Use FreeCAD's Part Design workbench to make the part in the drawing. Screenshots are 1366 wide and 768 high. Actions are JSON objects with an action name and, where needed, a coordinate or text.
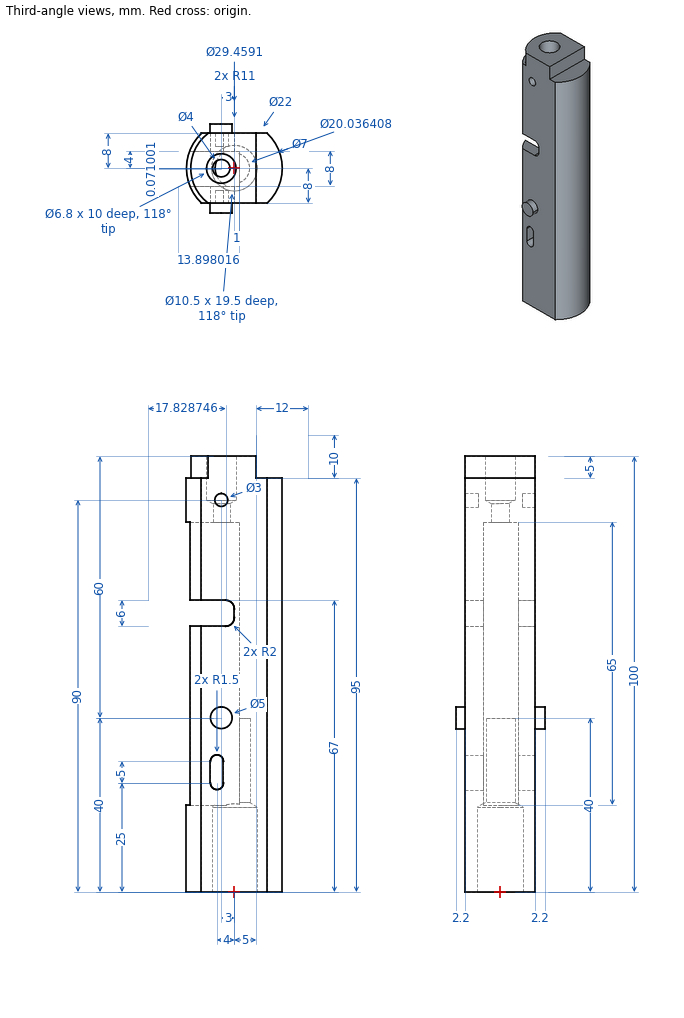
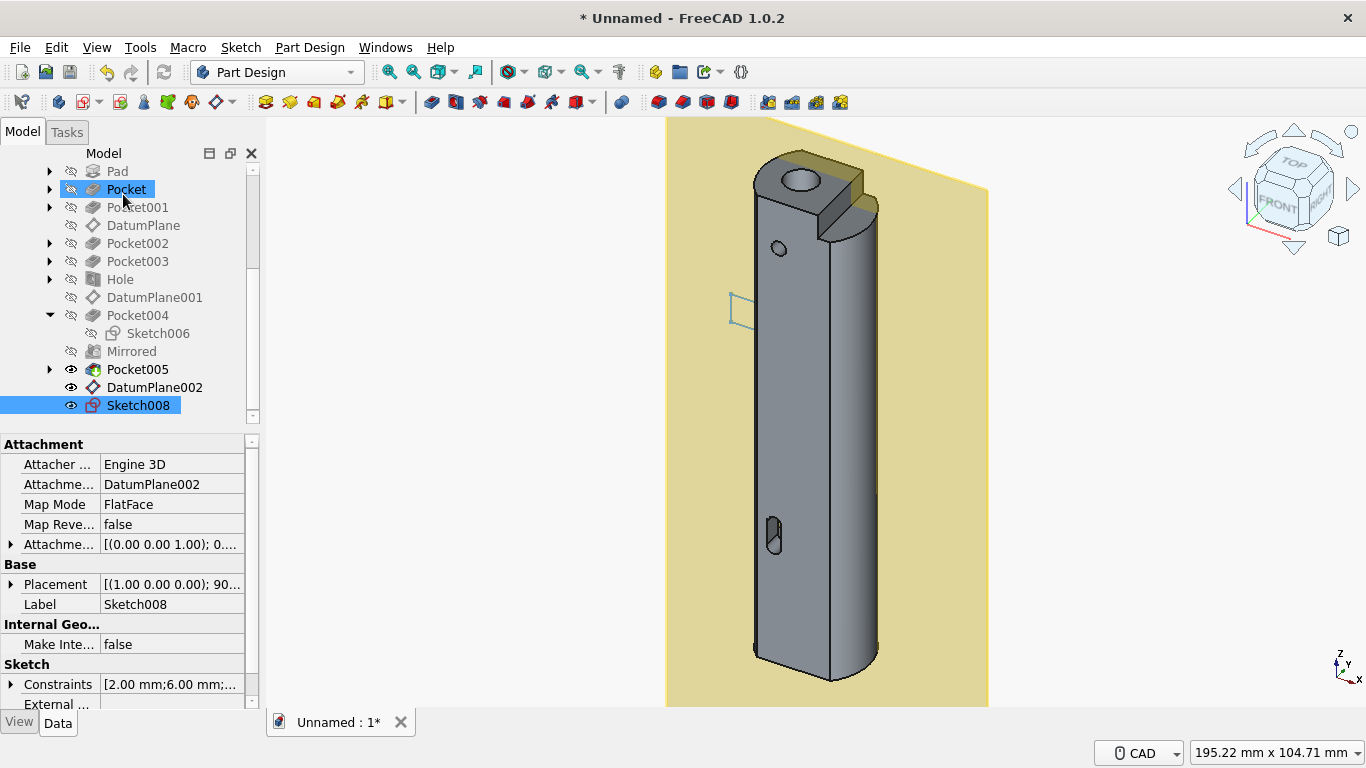
{"action": "left_click", "coordinate": [432, 102]}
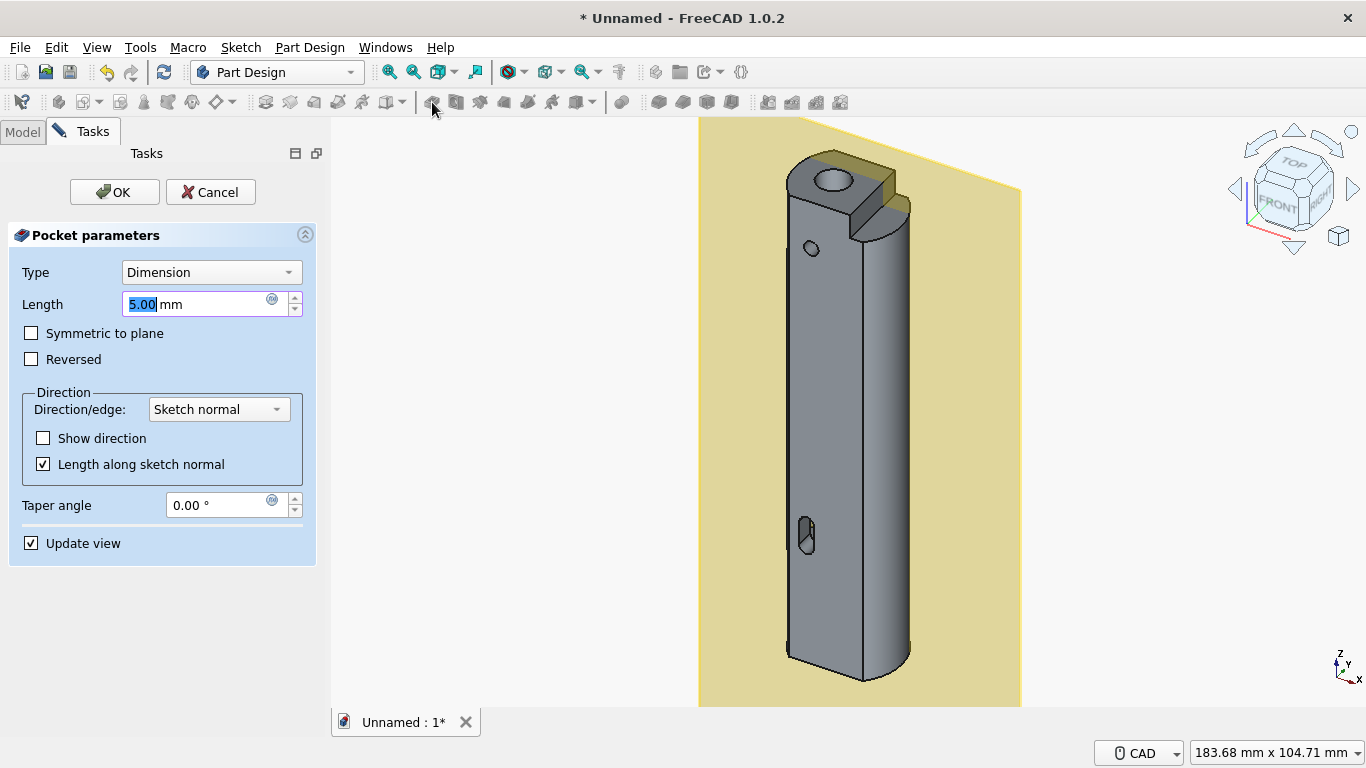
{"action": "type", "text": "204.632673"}
{"action": "key", "text": "Tab"}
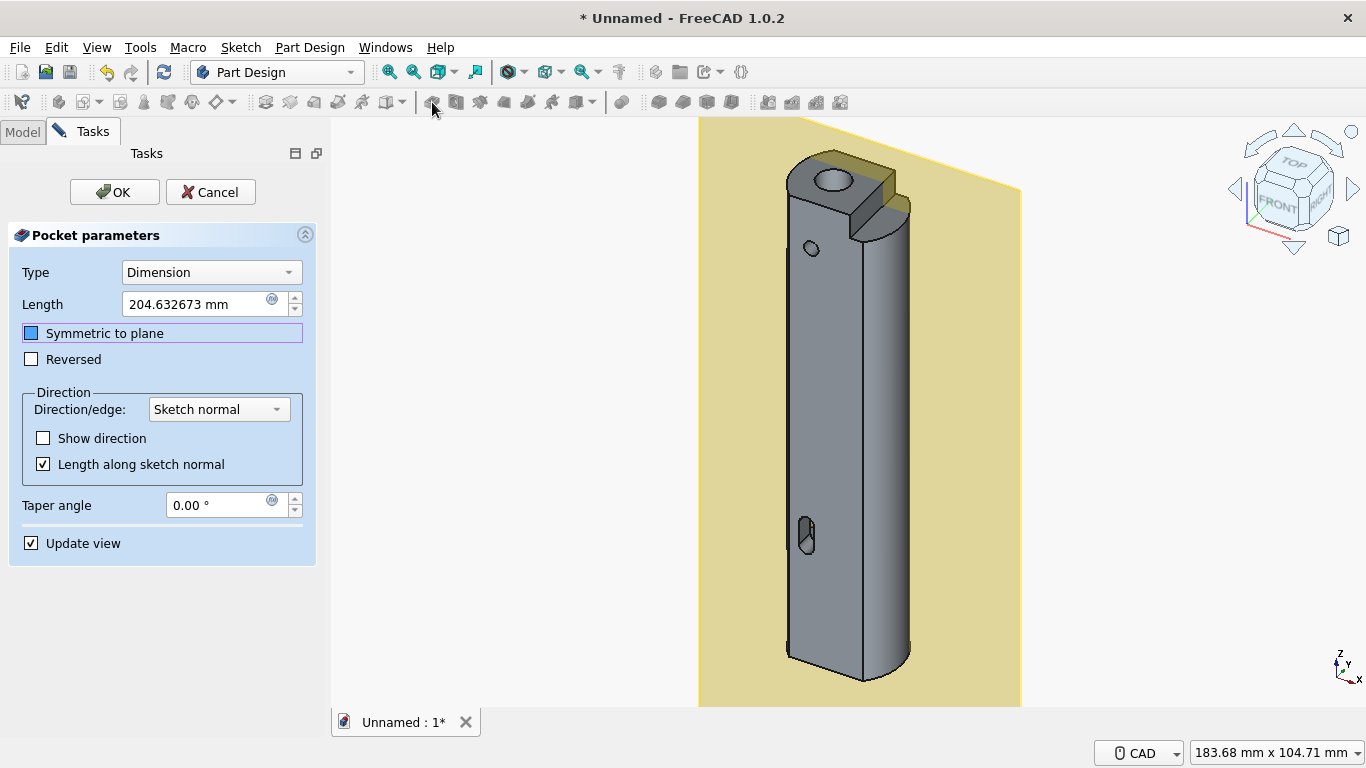
{"action": "left_click", "coordinate": [30, 333]}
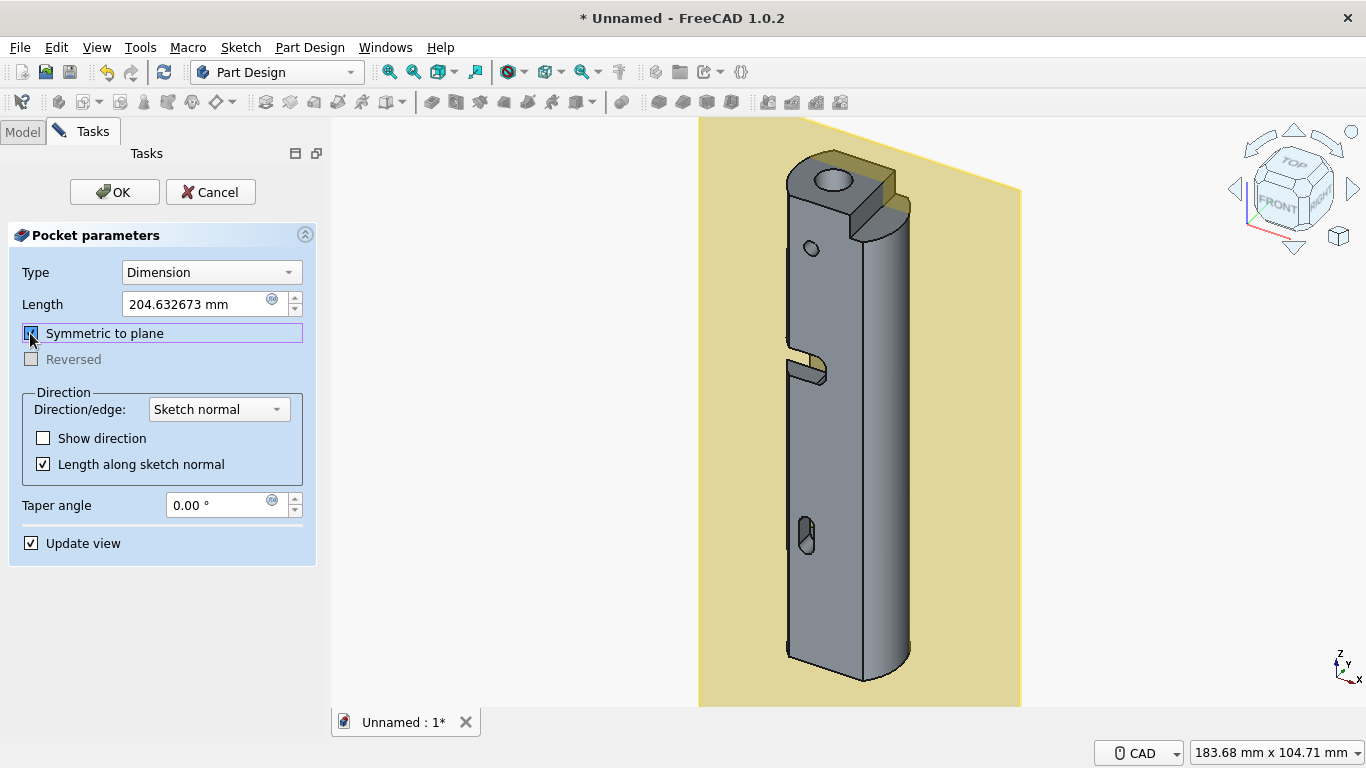
{"action": "left_click", "coordinate": [115, 192]}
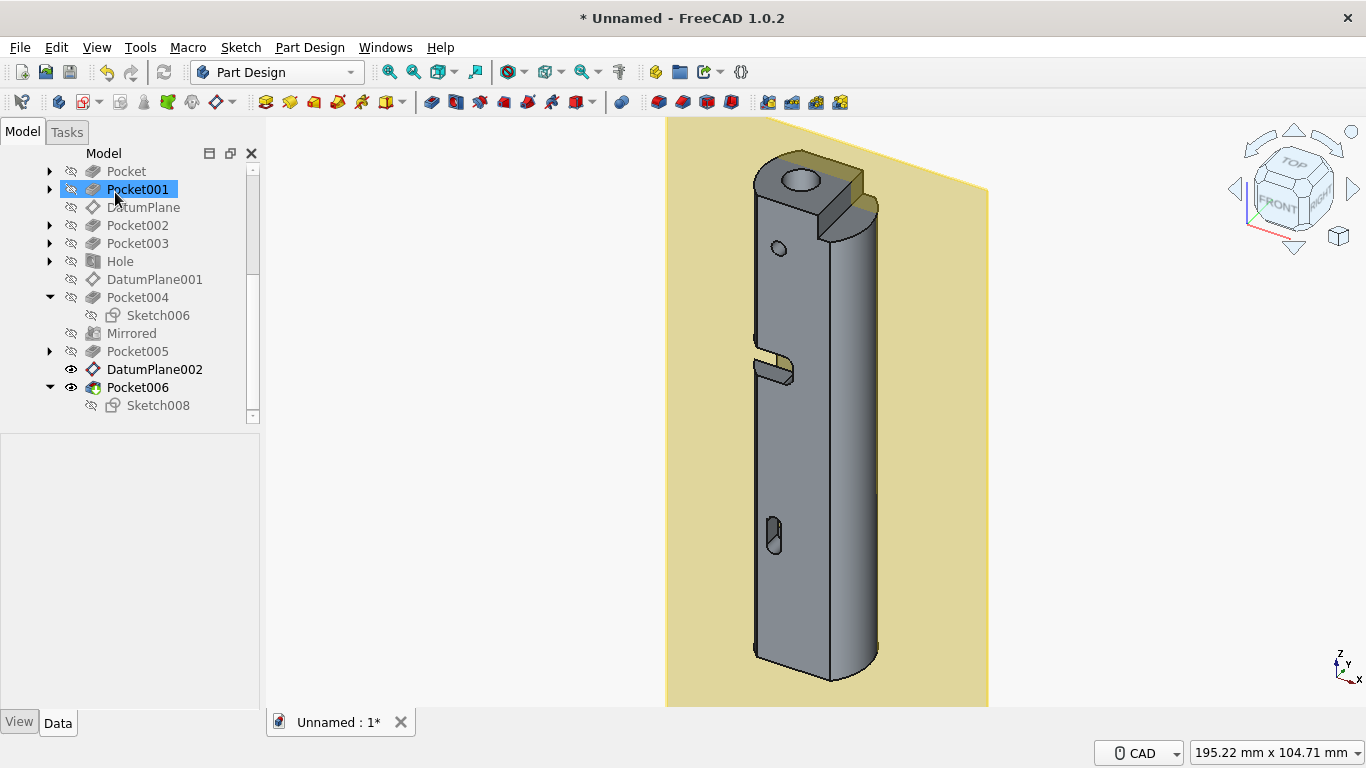
{"action": "left_click", "coordinate": [116, 369]}
{"action": "key", "text": "space"}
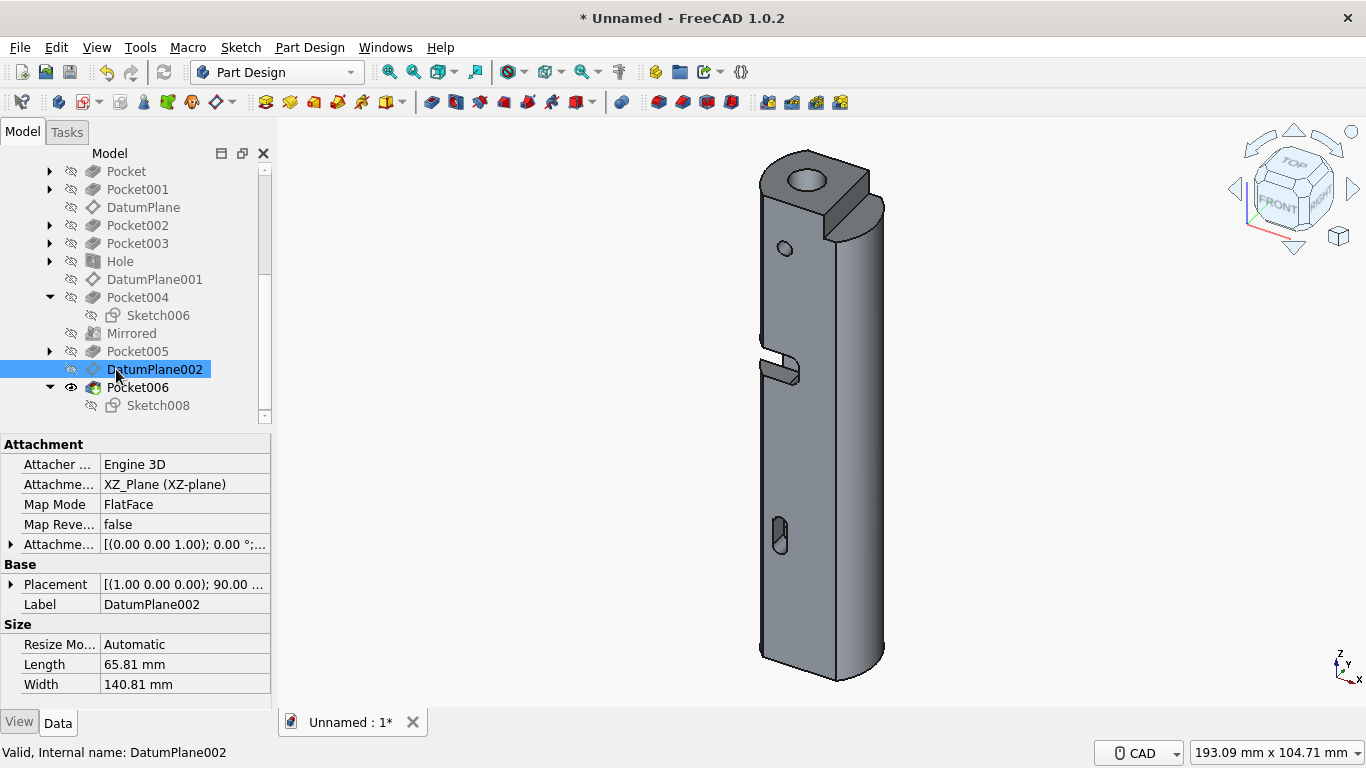
{"action": "left_click", "coordinate": [318, 667]}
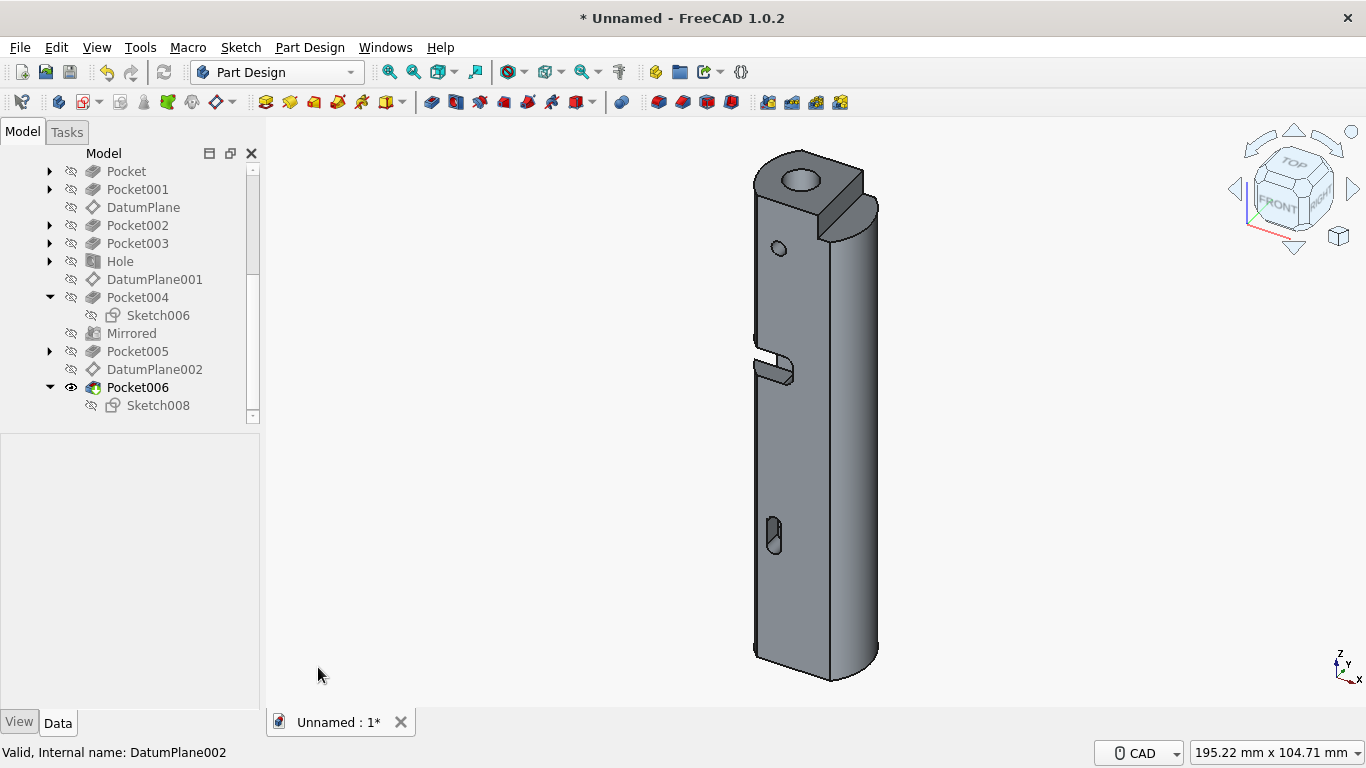
{"action": "left_click", "coordinate": [84, 102]}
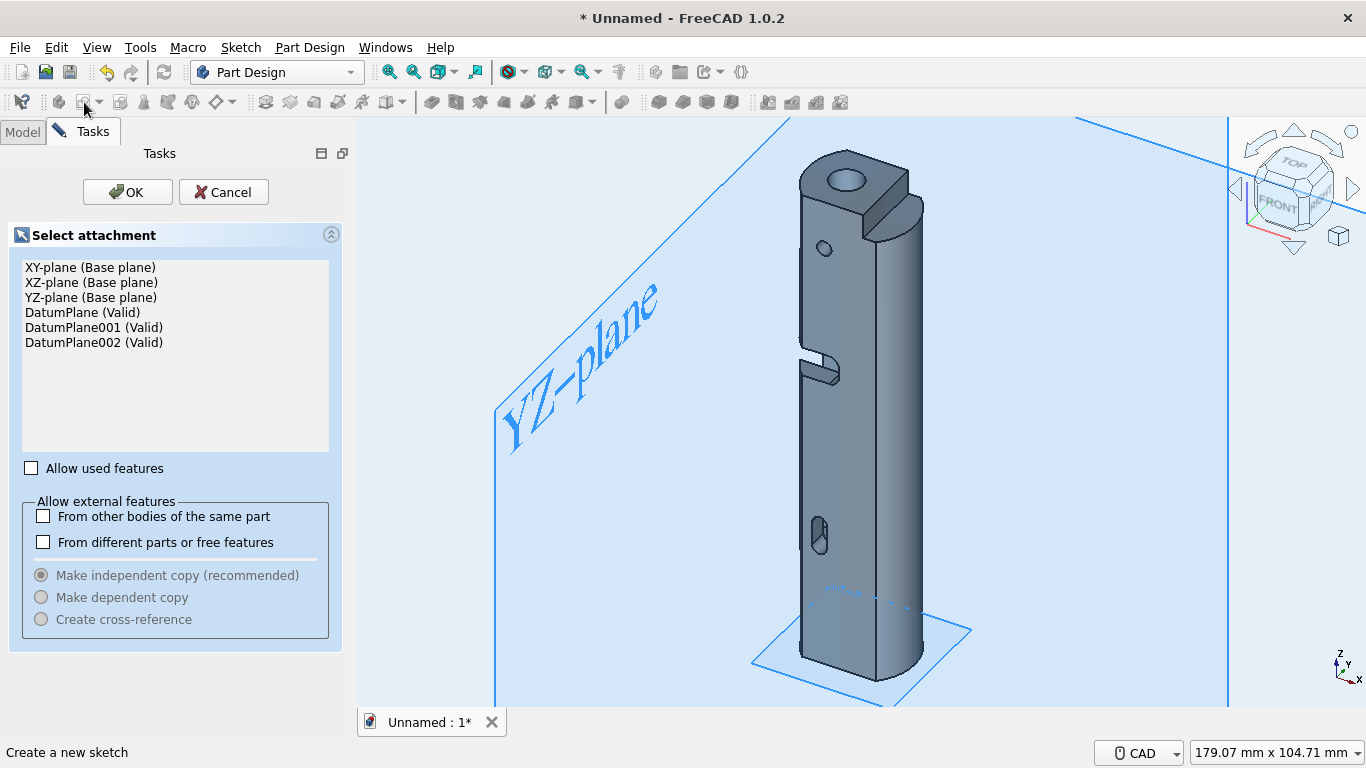
{"action": "left_click", "coordinate": [82, 268]}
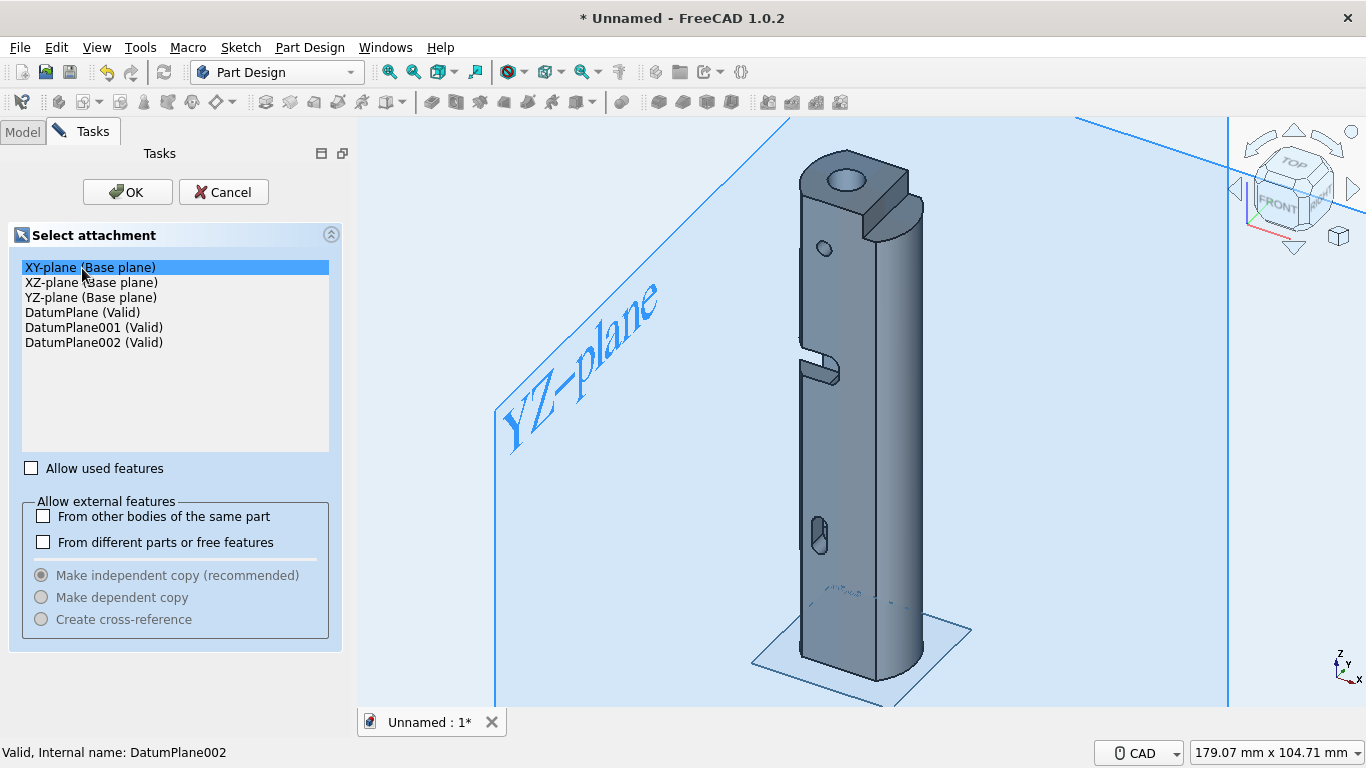
{"action": "left_click", "coordinate": [128, 192]}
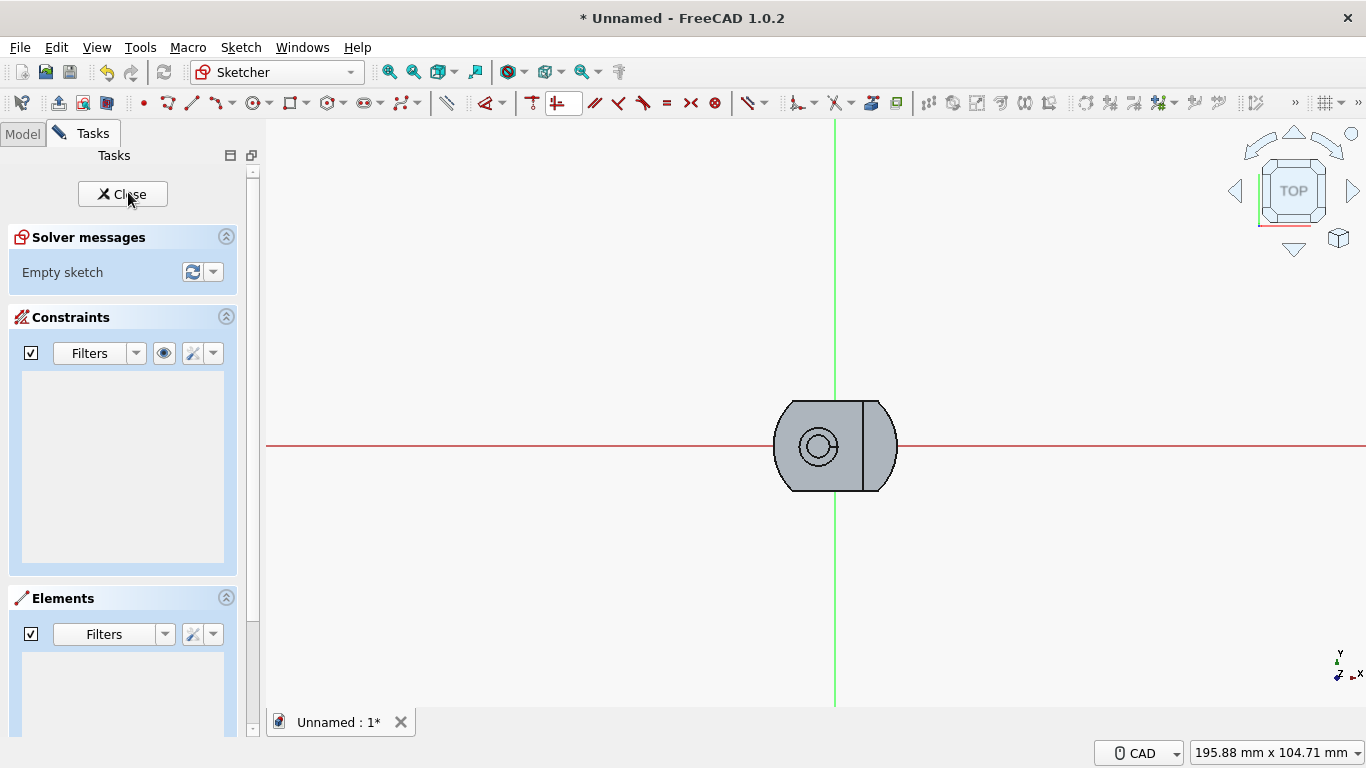
{"action": "key", "text": "q s"}